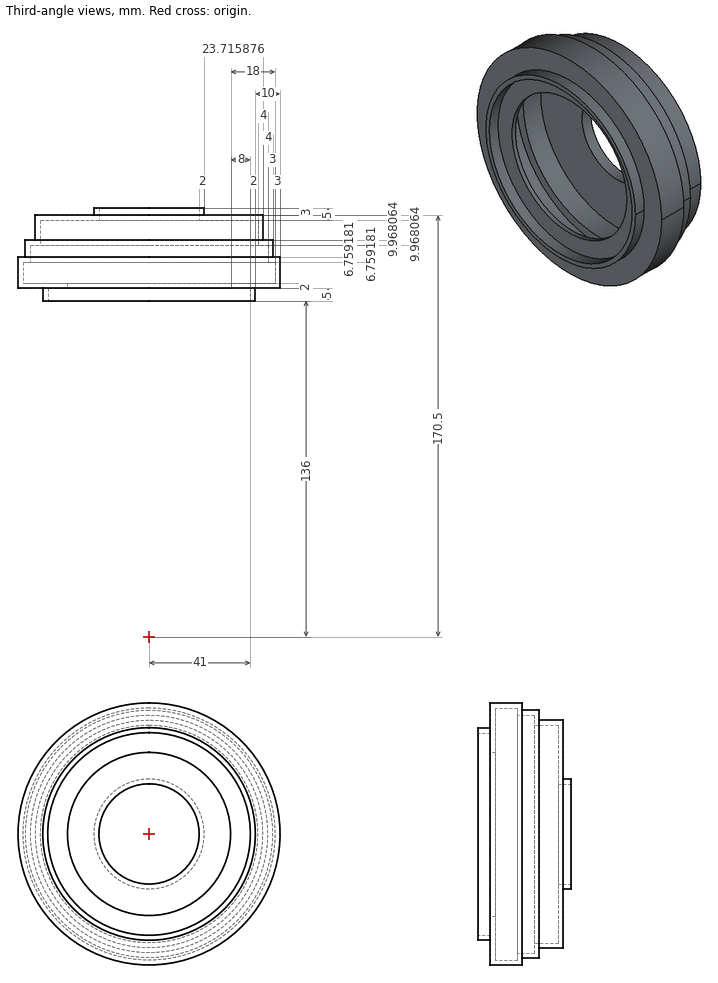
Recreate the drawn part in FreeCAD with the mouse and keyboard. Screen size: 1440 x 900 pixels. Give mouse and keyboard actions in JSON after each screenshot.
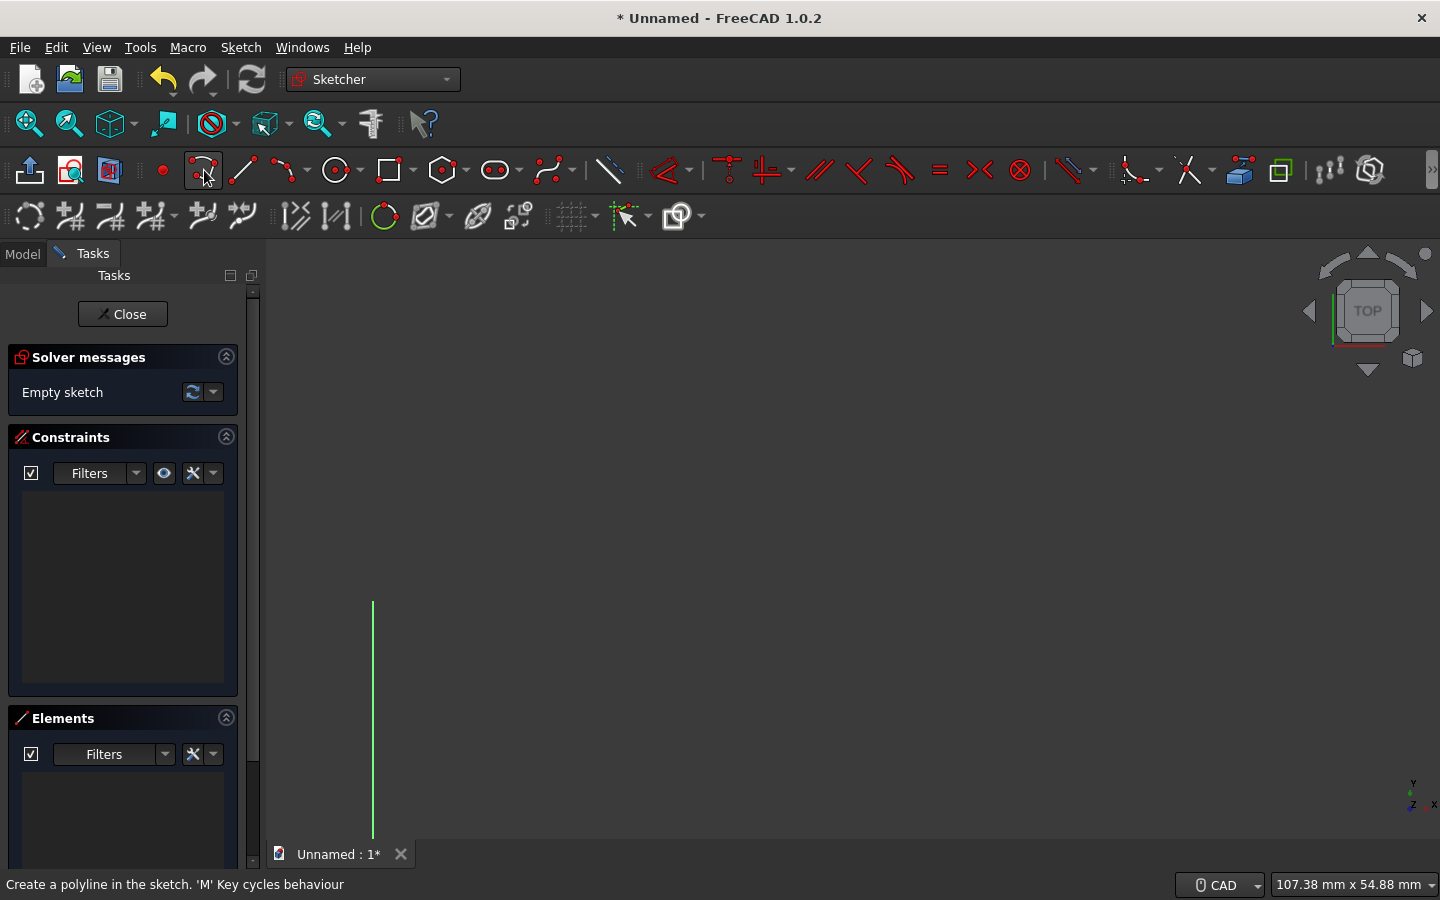
{"action": "left_click", "coordinate": [821, 737]}
{"action": "left_click", "coordinate": [843, 737]}
{"action": "left_click", "coordinate": [843, 682]}
{"action": "left_click", "coordinate": [952, 682]}
{"action": "left_click", "coordinate": [952, 543]}
{"action": "left_click", "coordinate": [920, 543]}
{"action": "left_click", "coordinate": [920, 469]}
{"action": "left_click", "coordinate": [876, 469]}
{"action": "left_click", "coordinate": [876, 360]}
{"action": "left_click", "coordinate": [617, 360]}
{"action": "left_click", "coordinate": [617, 327]}
{"action": "left_click", "coordinate": [595, 327]}
{"action": "left_click", "coordinate": [595, 382]}
{"action": "left_click", "coordinate": [854, 382]}
{"action": "left_click", "coordinate": [854, 491]}
{"action": "left_click", "coordinate": [898, 491]}
{"action": "left_click", "coordinate": [898, 565]}
{"action": "left_click", "coordinate": [931, 565]}
{"action": "left_click", "coordinate": [931, 661]}
{"action": "left_click", "coordinate": [734, 661]}
{"action": "left_click", "coordinate": [734, 682]}
{"action": "left_click", "coordinate": [821, 682]}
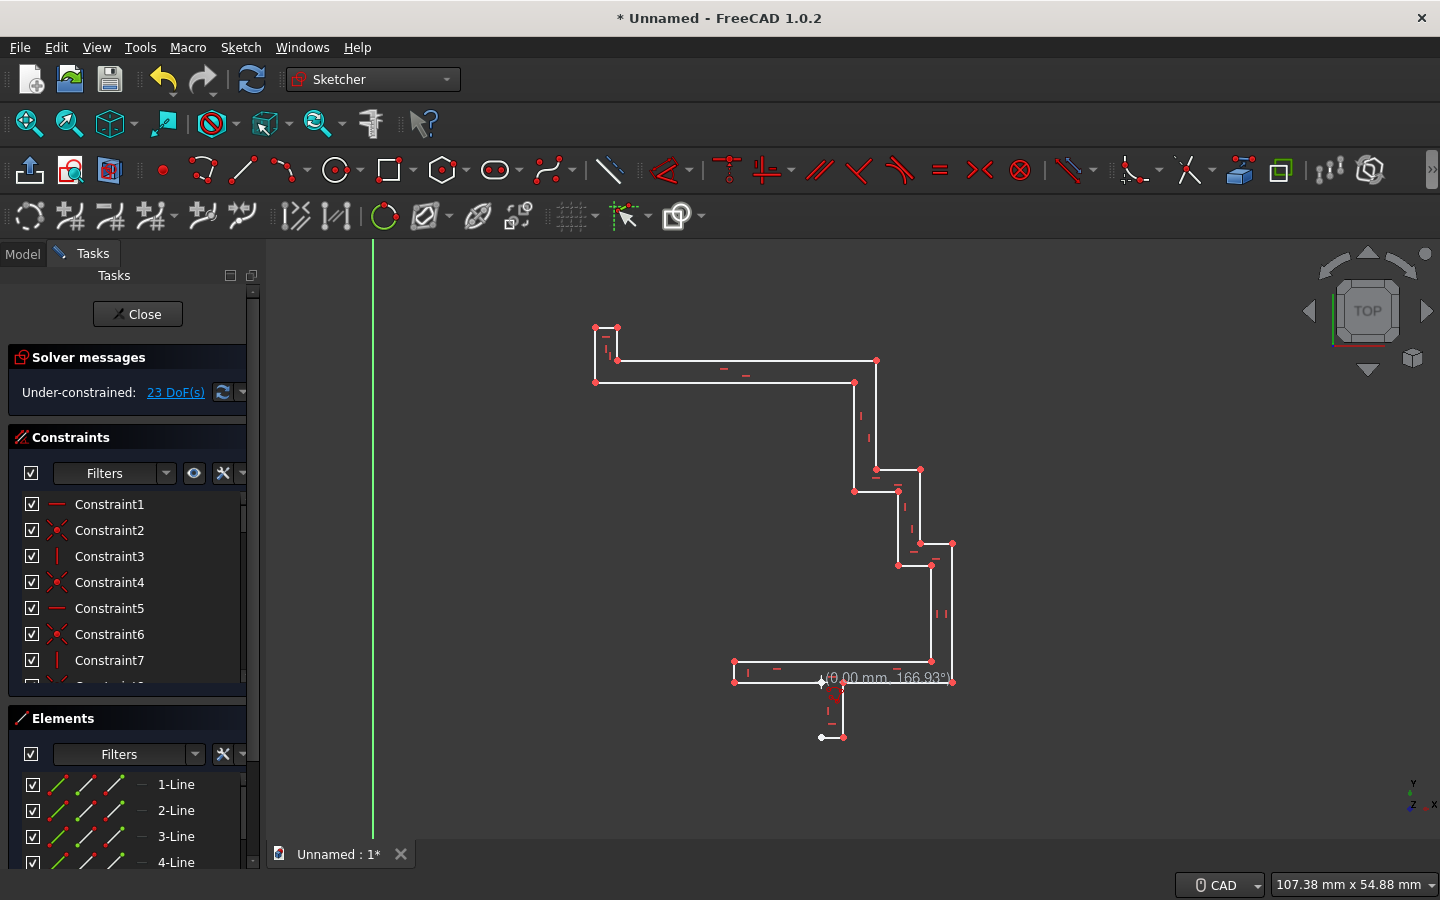
{"action": "scroll", "coordinate": [821, 737], "scroll_direction": "up", "scroll_amount": 2}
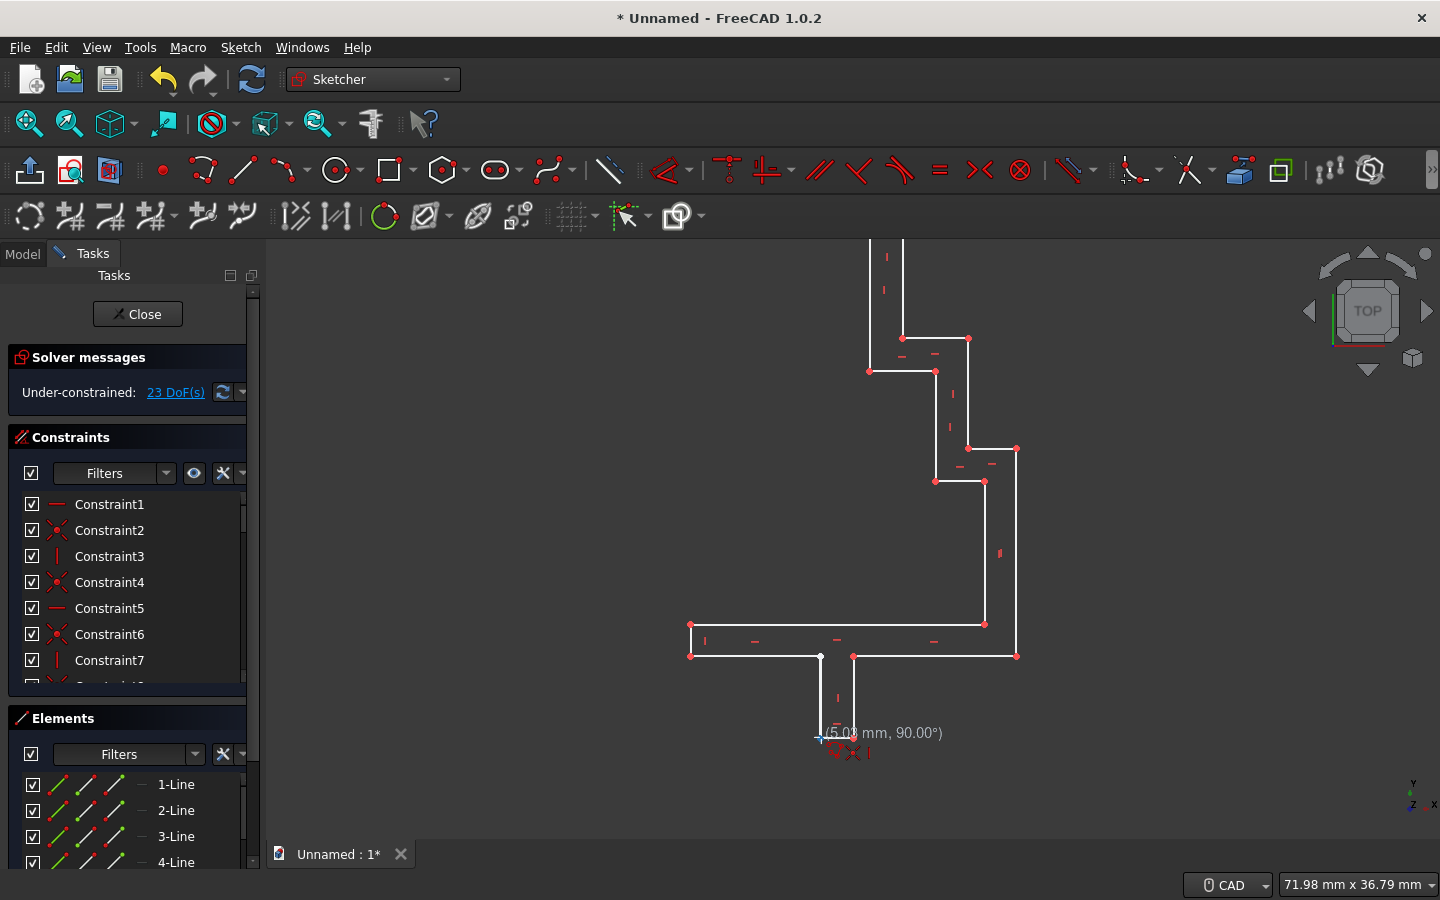
{"action": "left_click", "coordinate": [821, 738]}
{"action": "key", "text": "Escape"}
{"action": "key", "text": "Escape"}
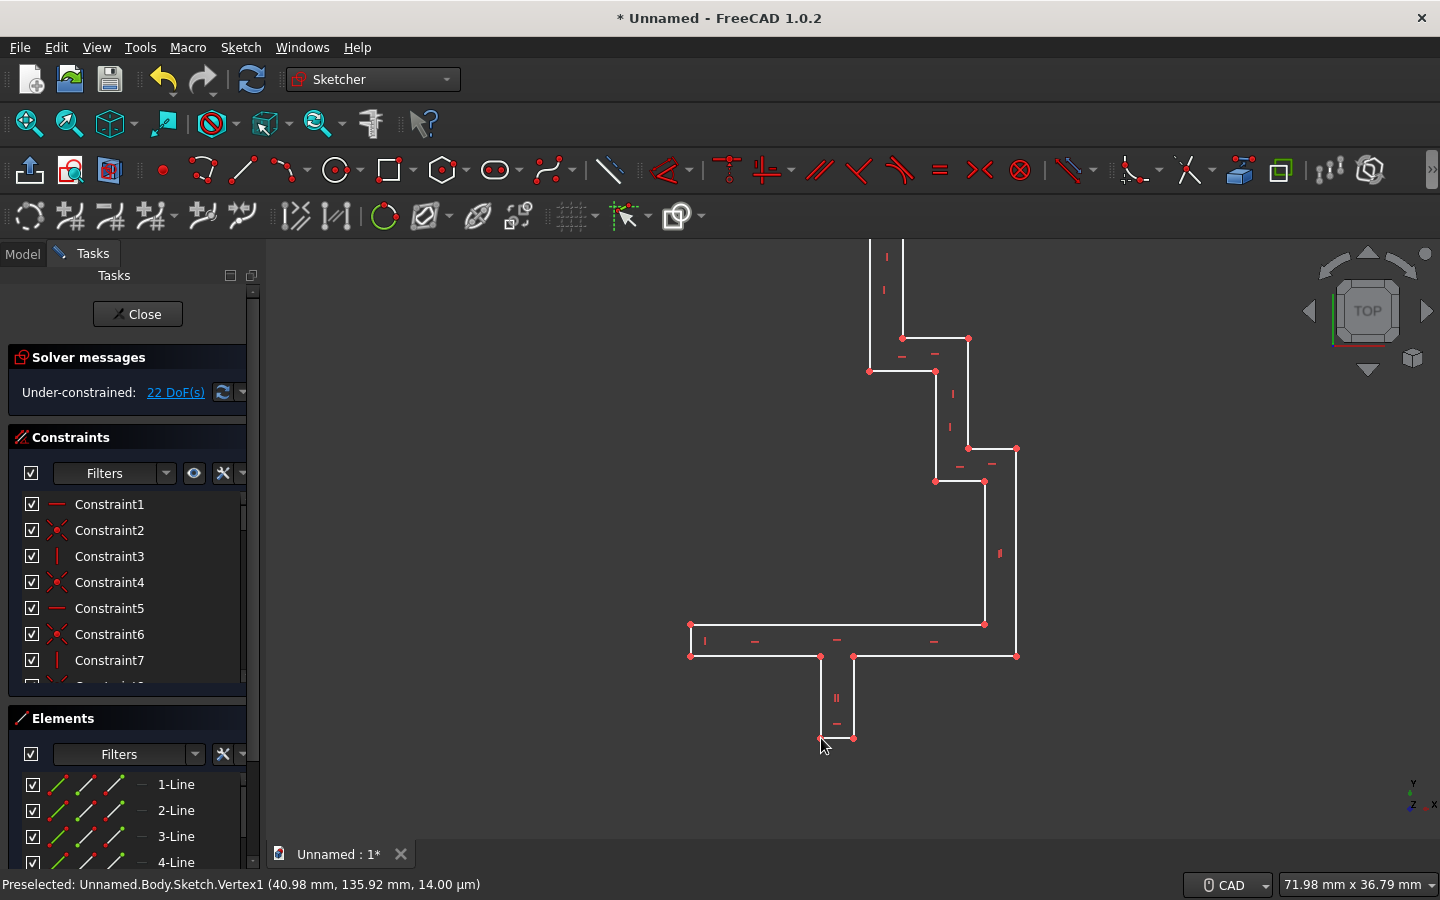
{"action": "left_click", "coordinate": [664, 170]}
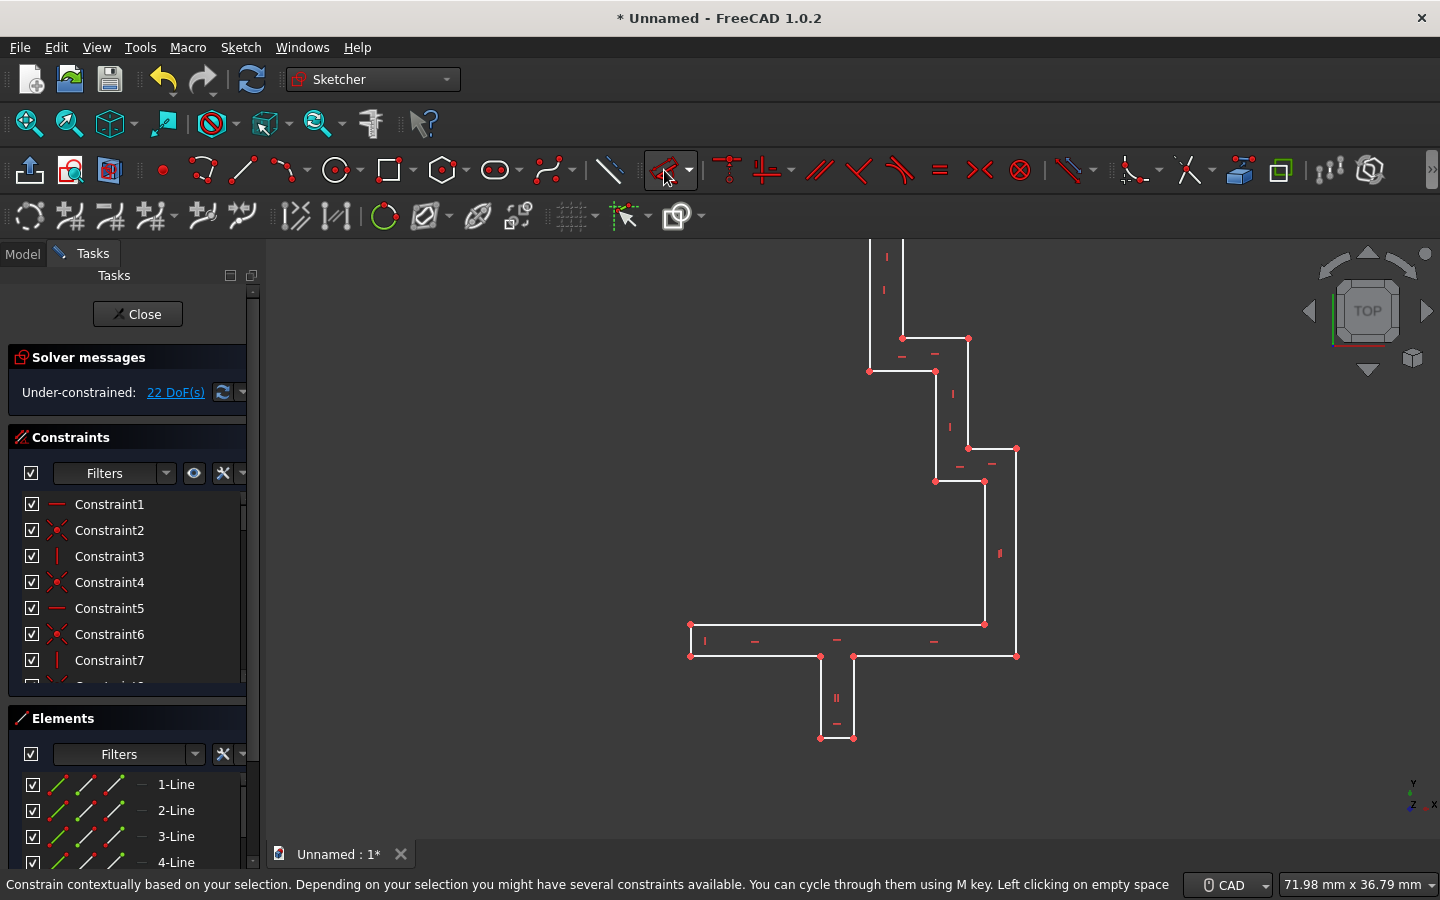
{"action": "scroll", "coordinate": [831, 738], "scroll_direction": "up", "scroll_amount": 2}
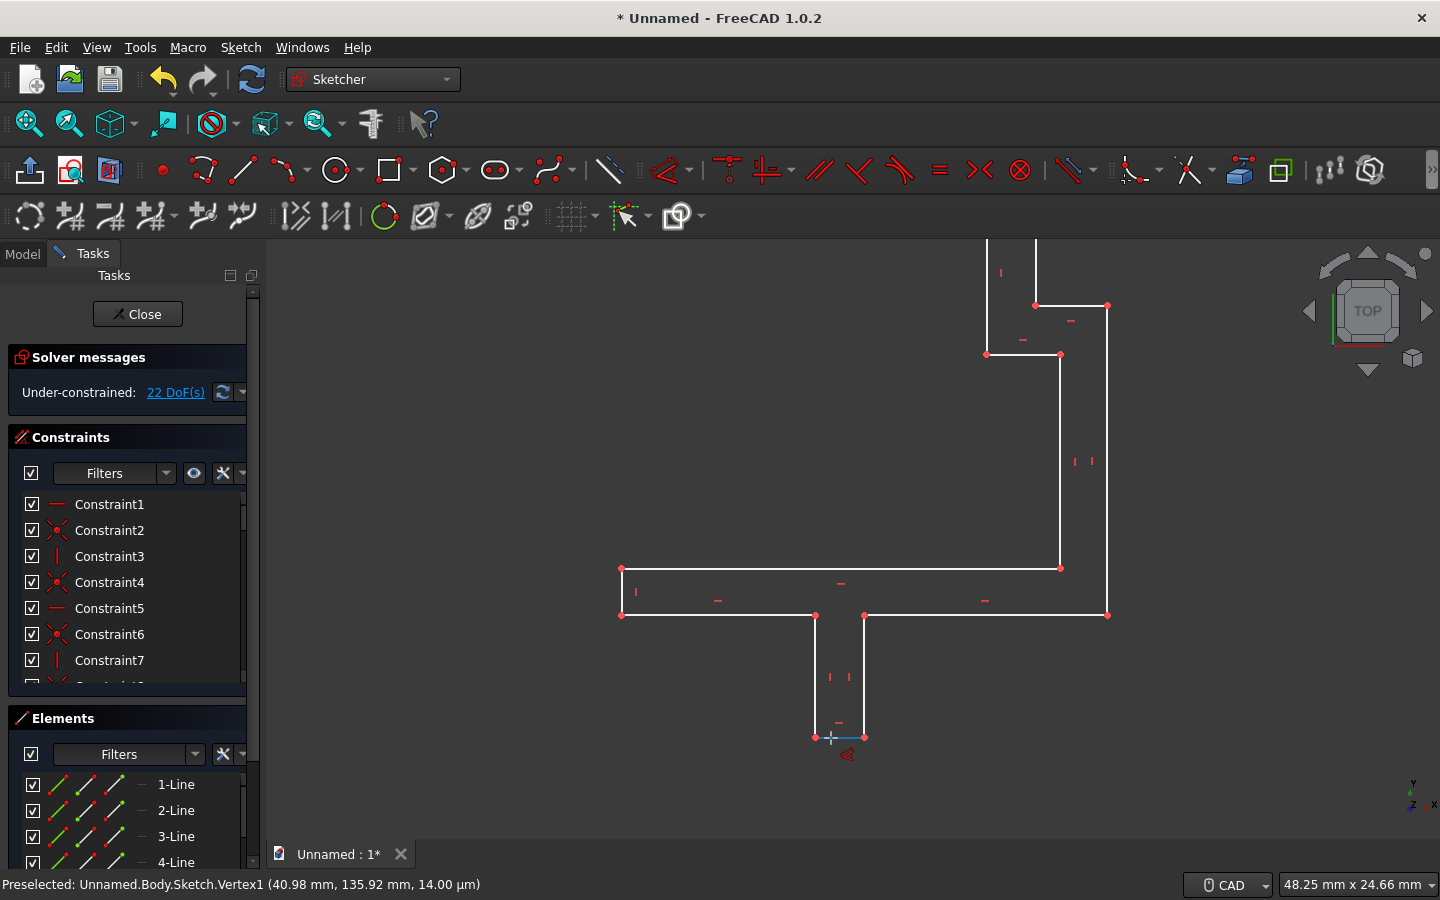
{"action": "left_click", "coordinate": [830, 738]}
{"action": "left_click", "coordinate": [840, 772]}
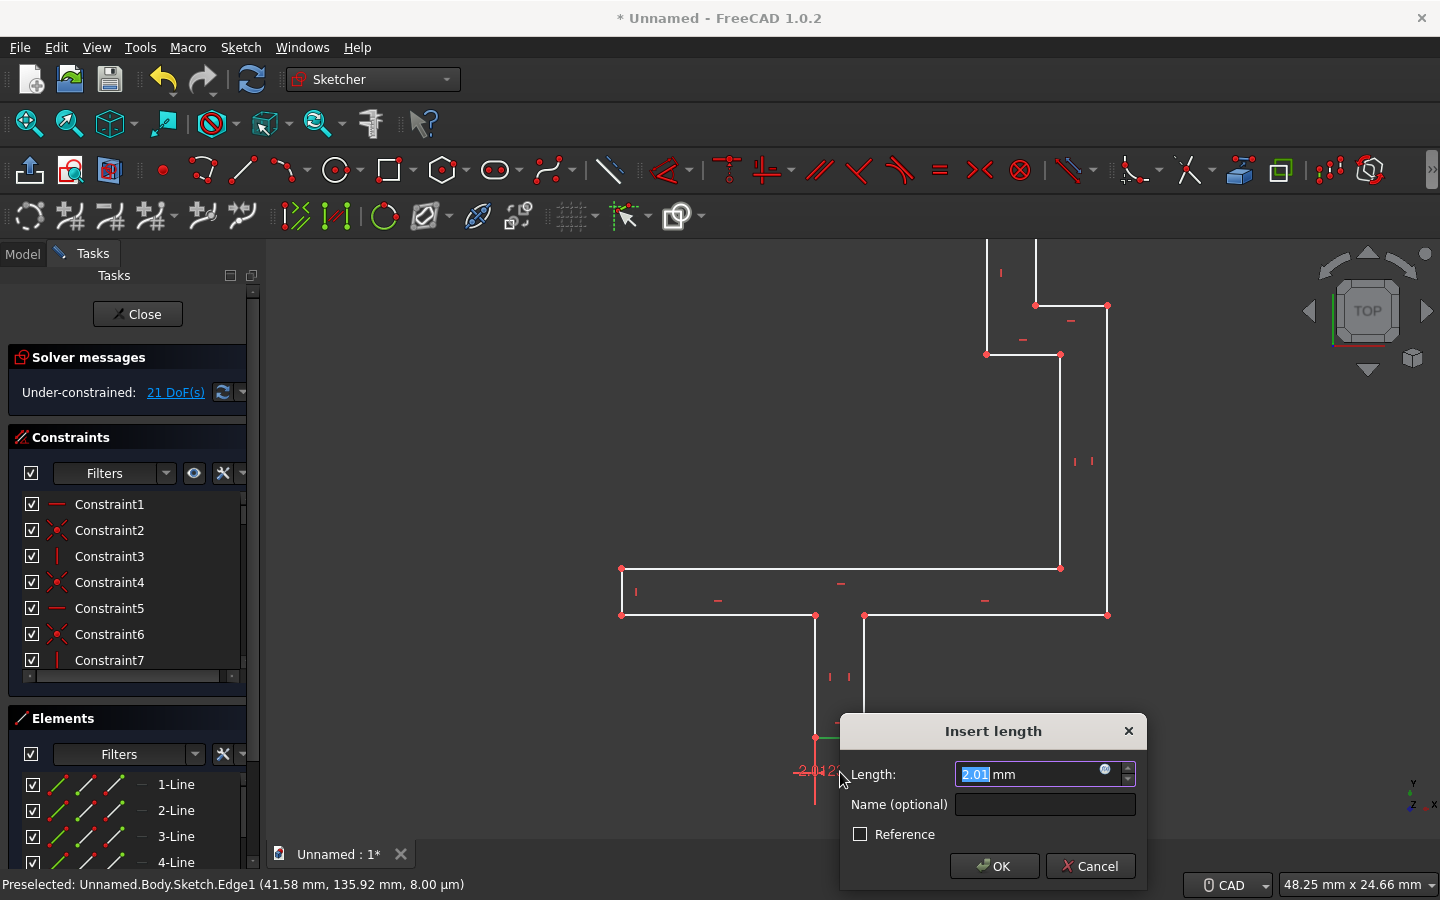
{"action": "type", "text": "2"}
{"action": "key", "text": "Return"}